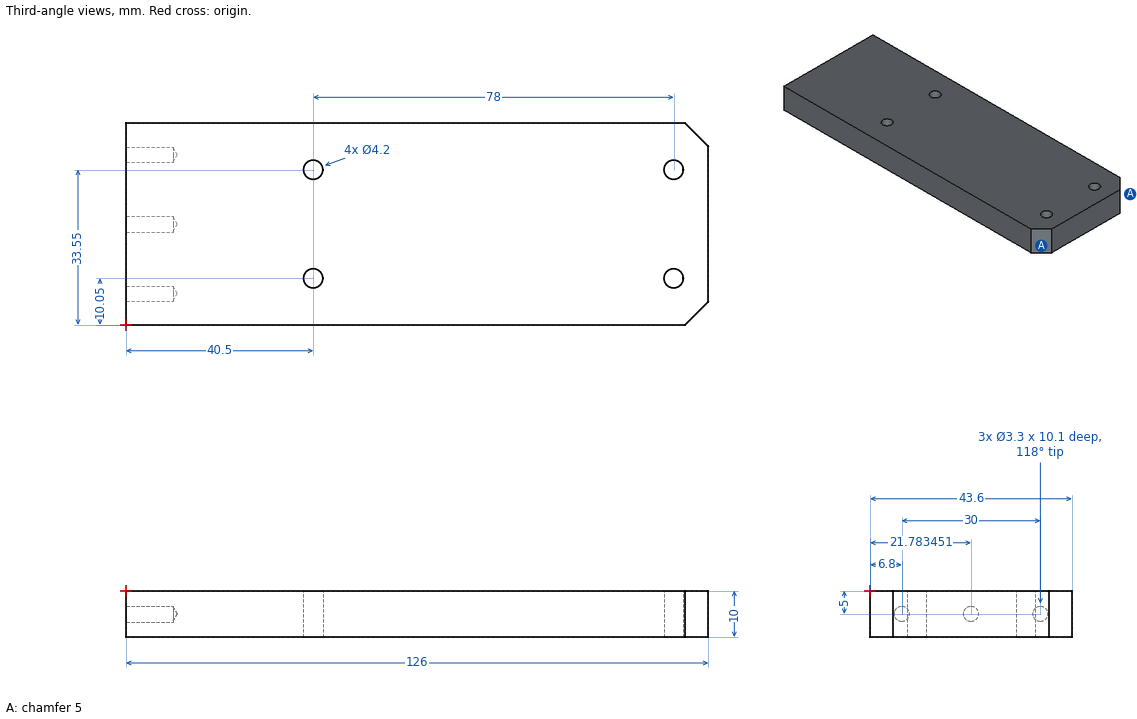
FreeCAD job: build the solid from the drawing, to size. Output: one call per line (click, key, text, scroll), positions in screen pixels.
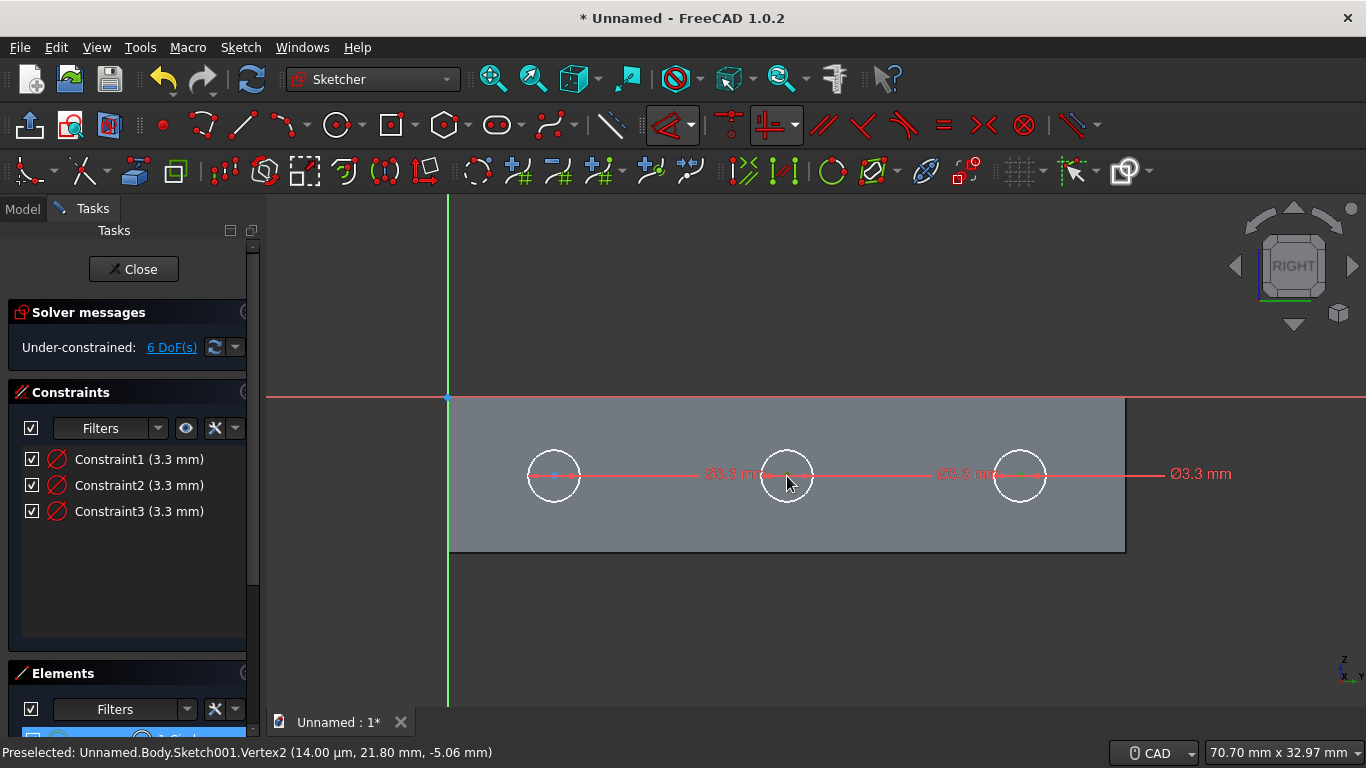
key(h)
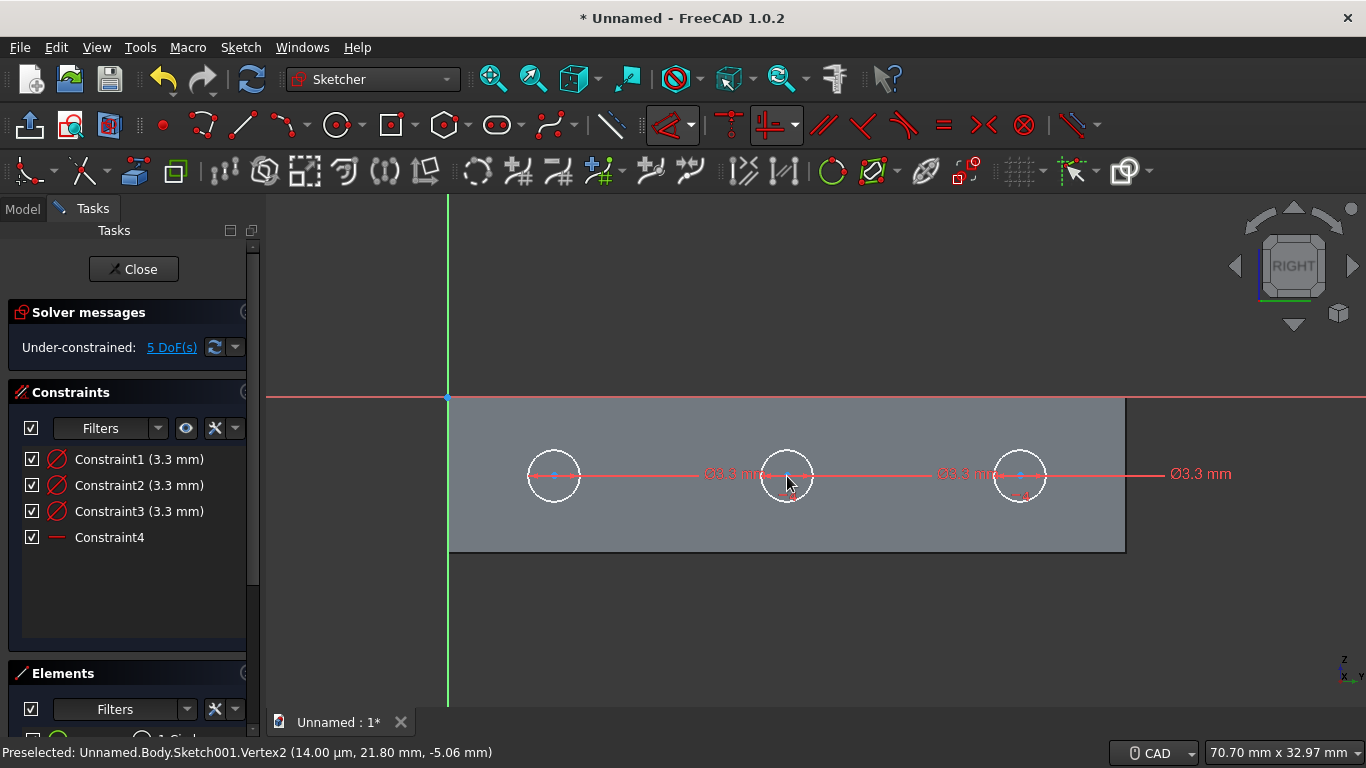
click(787, 476)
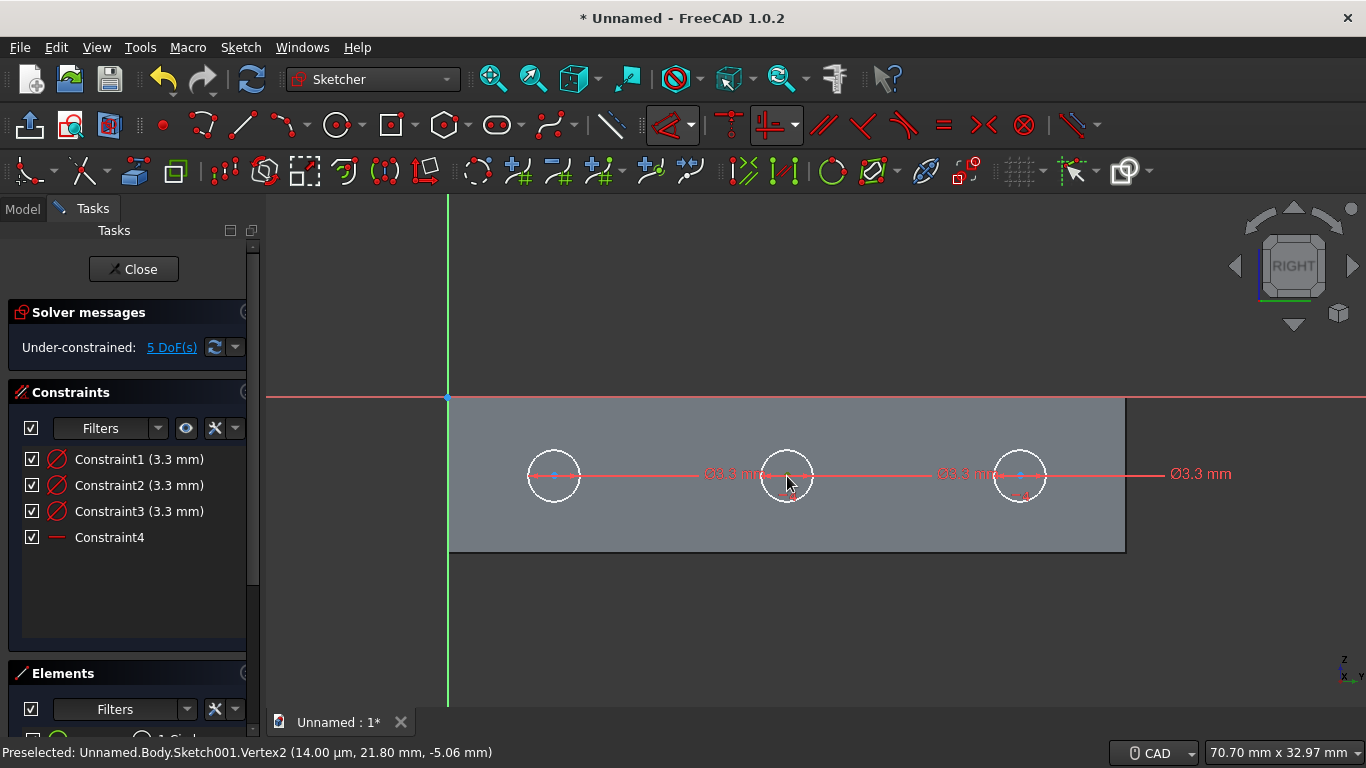
click(554, 476)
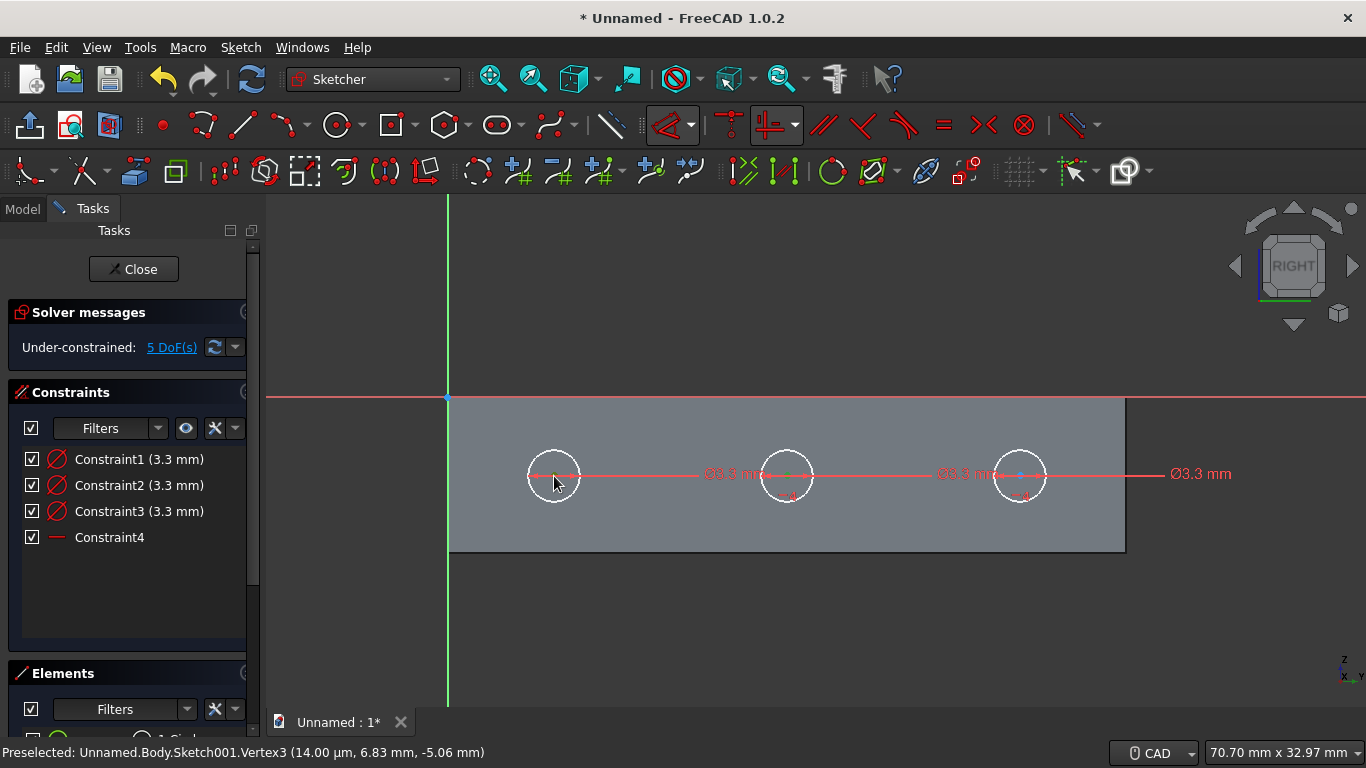
click(798, 126)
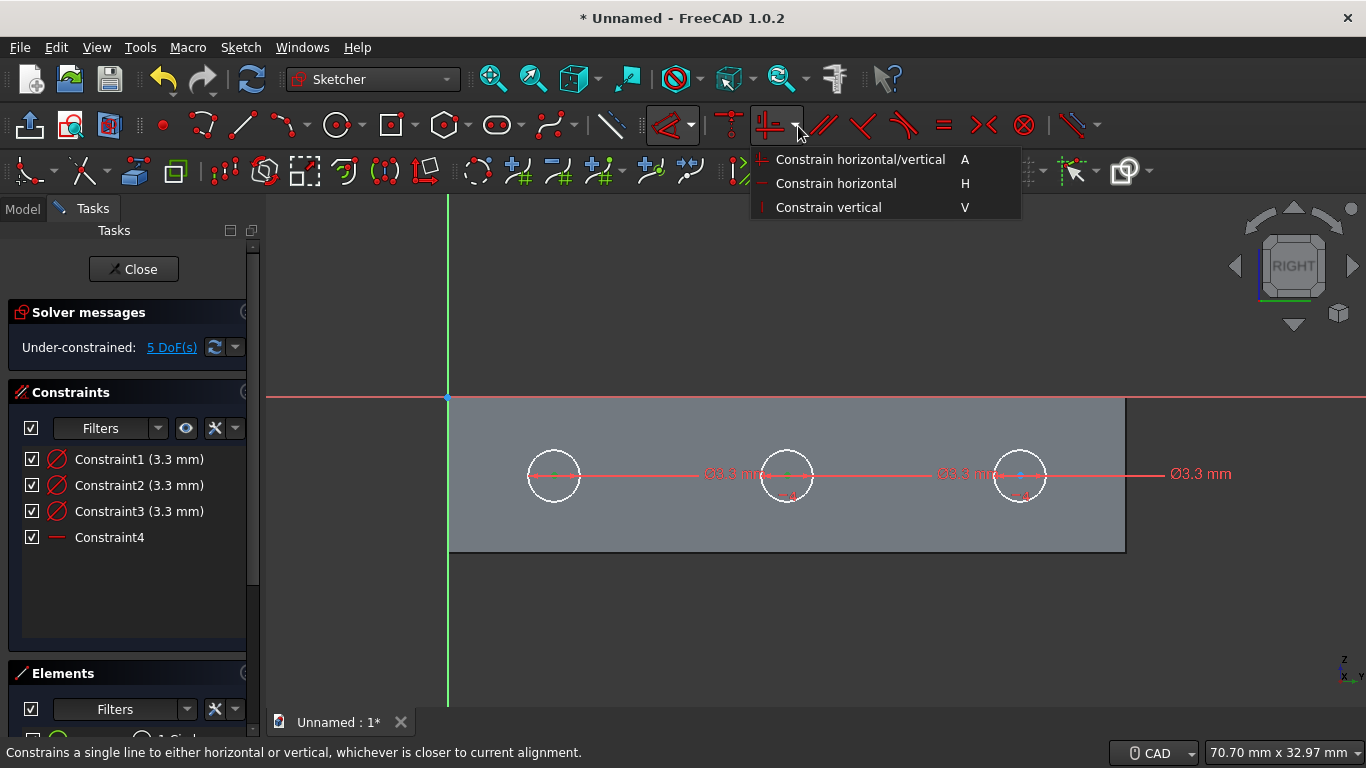
click(886, 183)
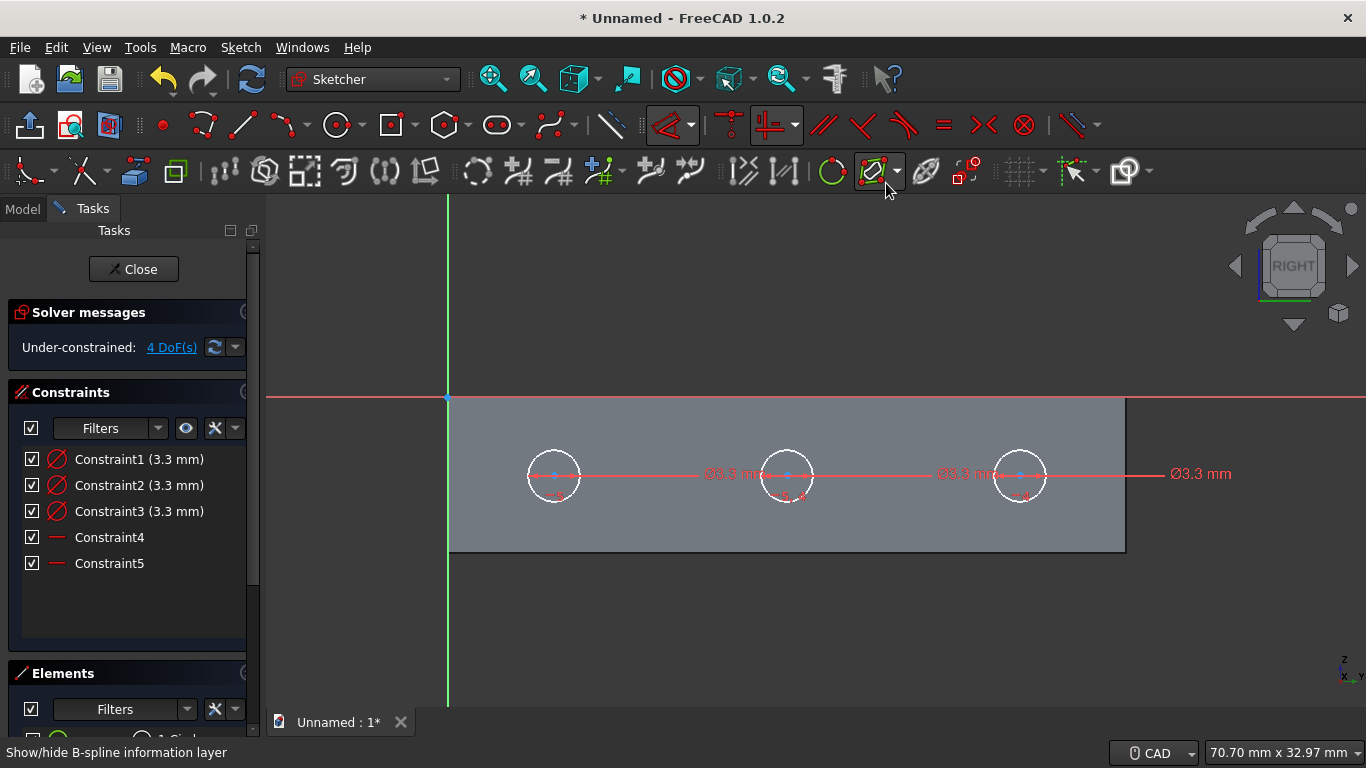
click(666, 126)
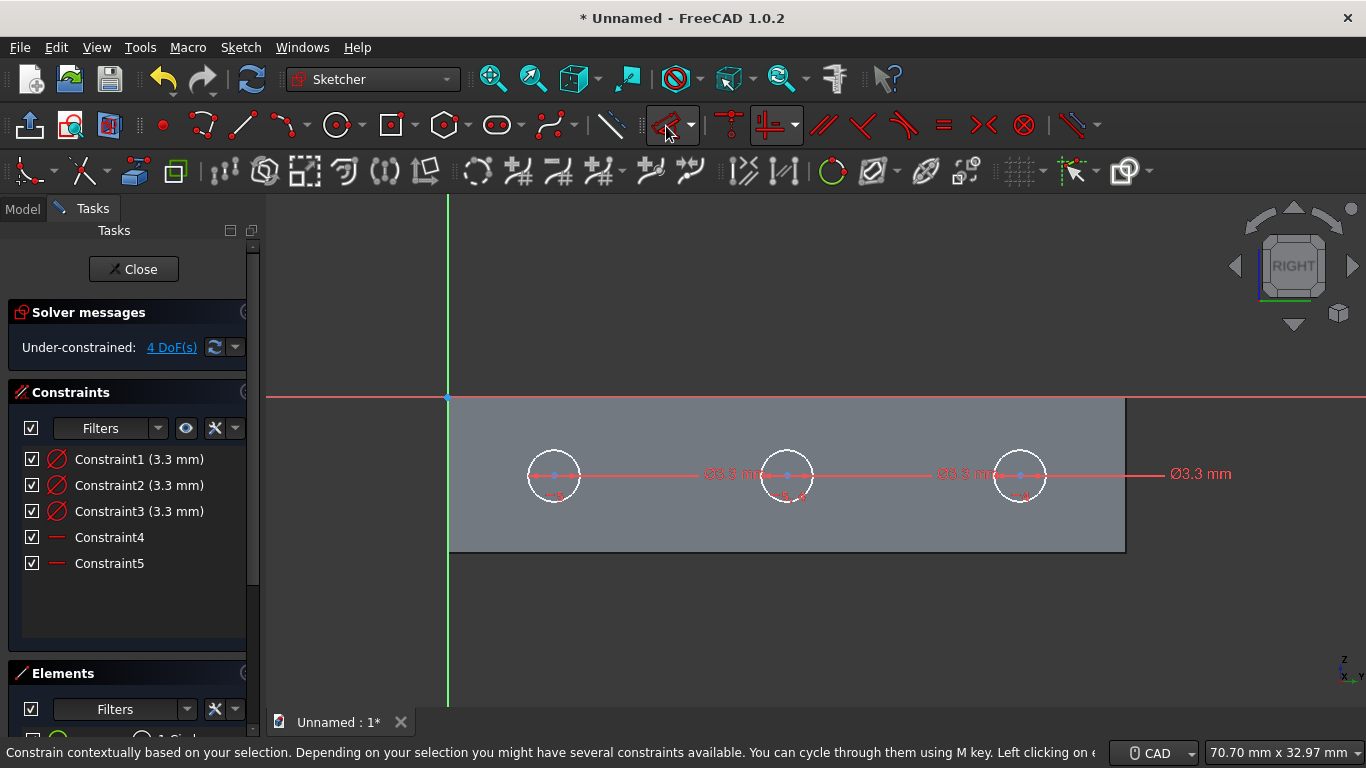
click(1020, 476)
click(414, 437)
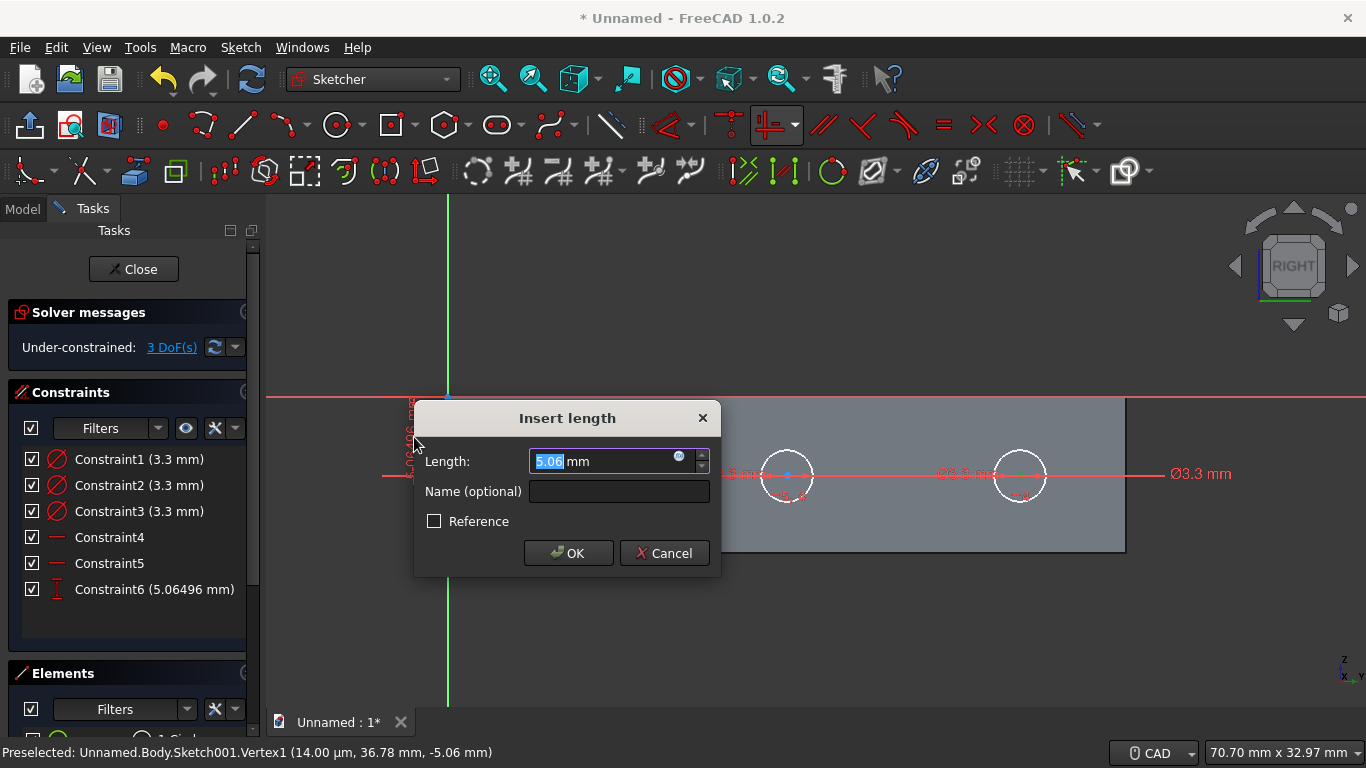
text(5)
key(Return)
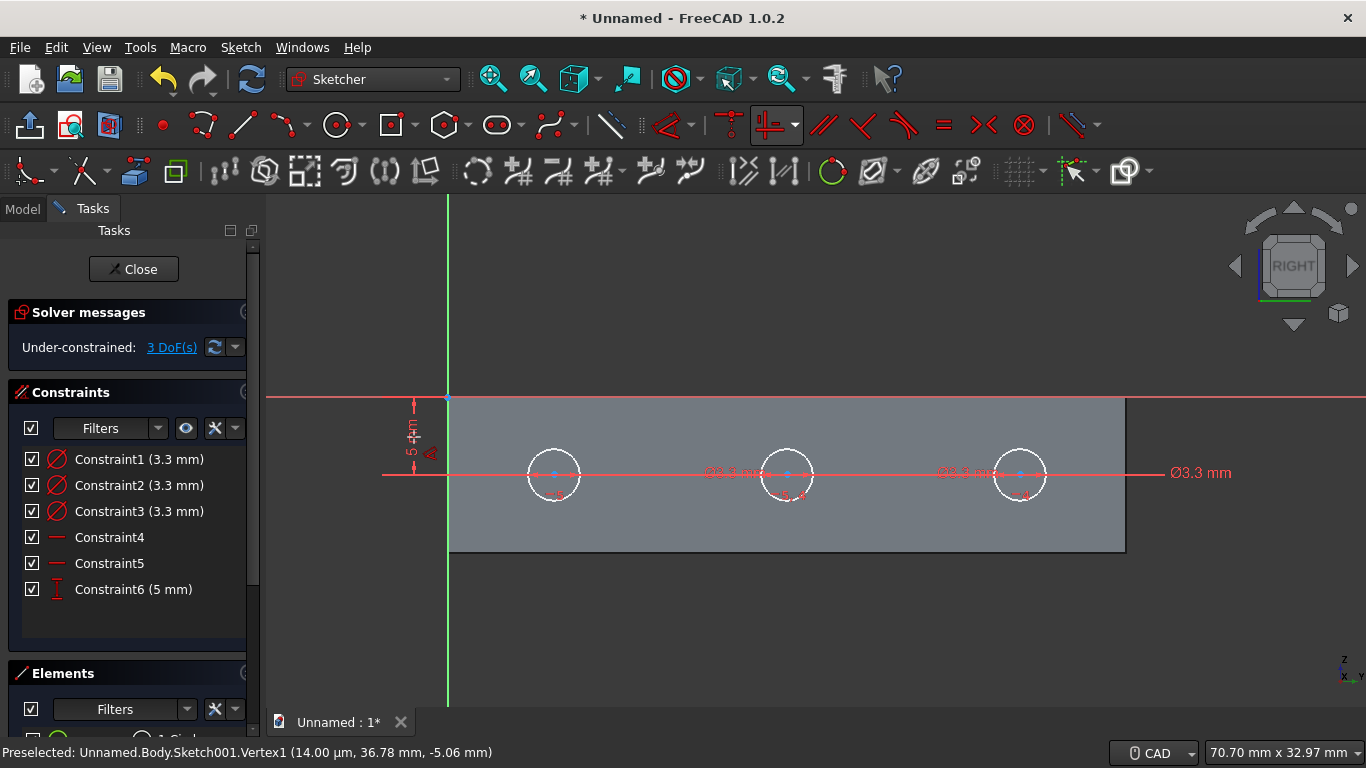
click(554, 475)
click(501, 363)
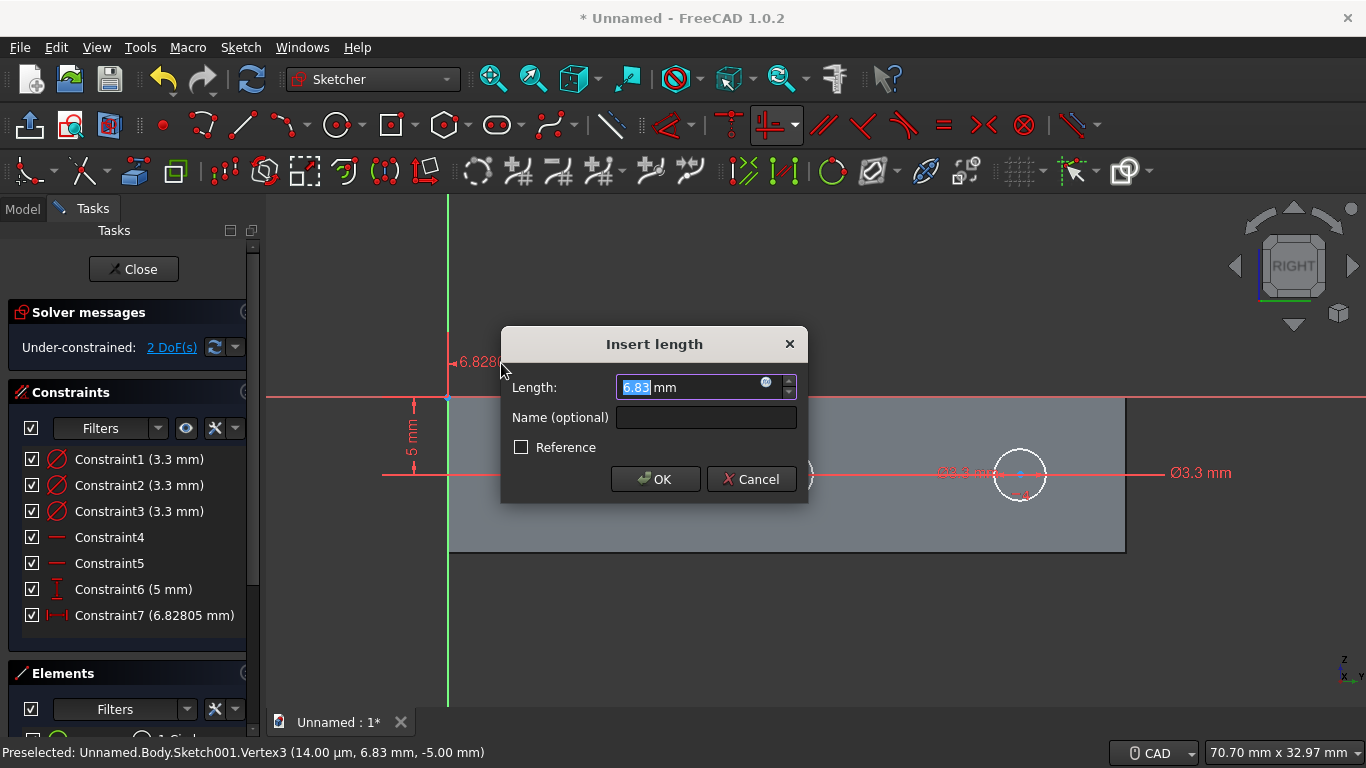
text(6.8)
key(Return)